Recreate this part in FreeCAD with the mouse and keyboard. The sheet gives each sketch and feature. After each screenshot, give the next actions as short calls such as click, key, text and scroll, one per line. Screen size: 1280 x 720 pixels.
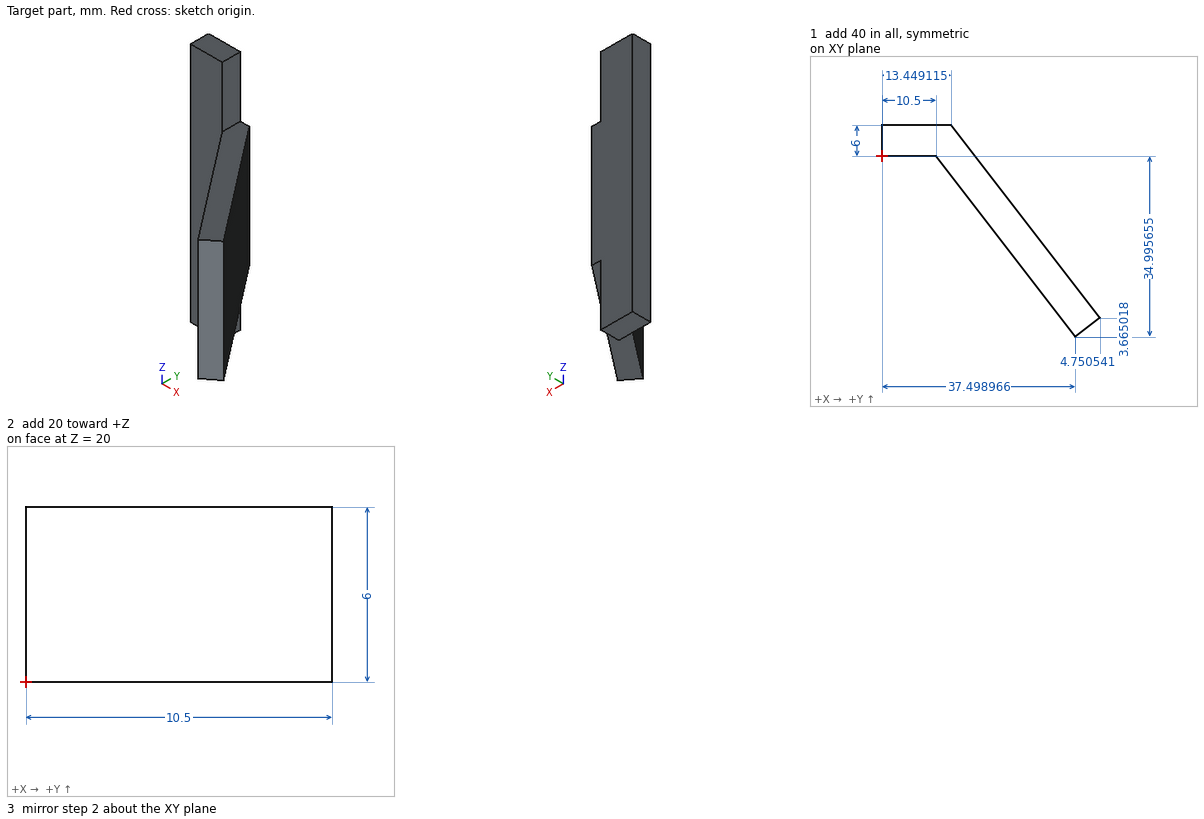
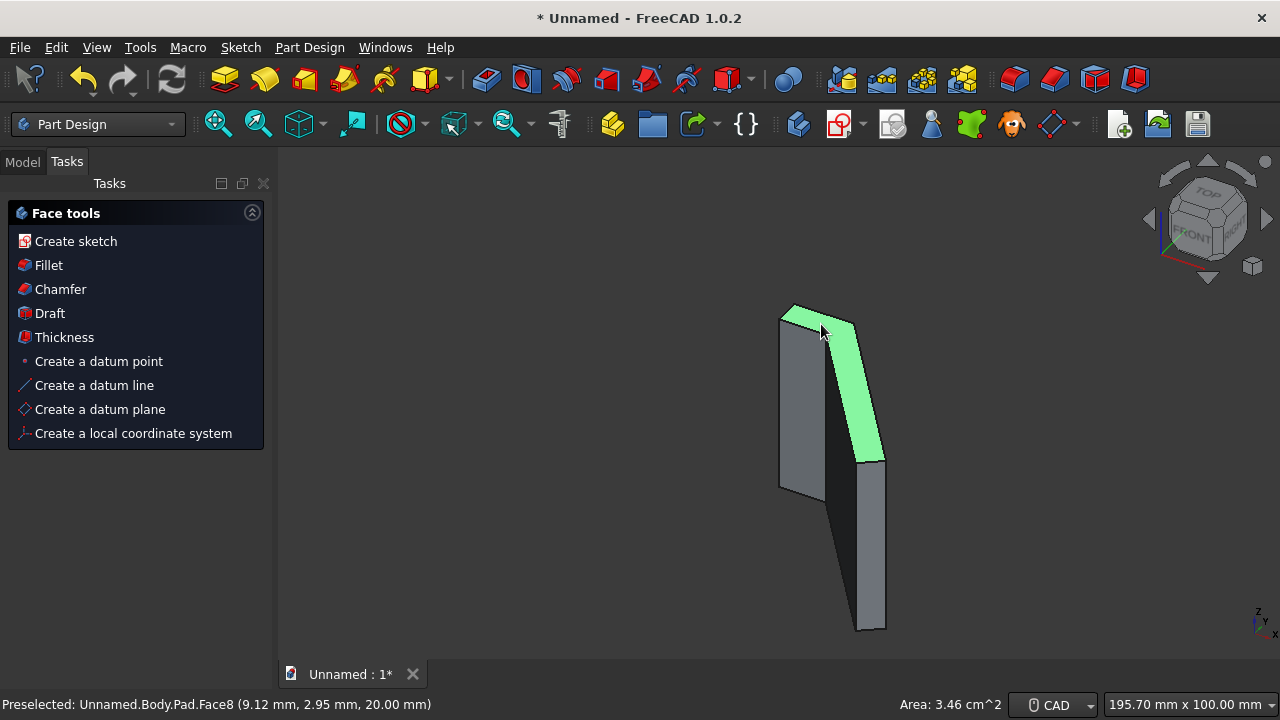
click(840, 124)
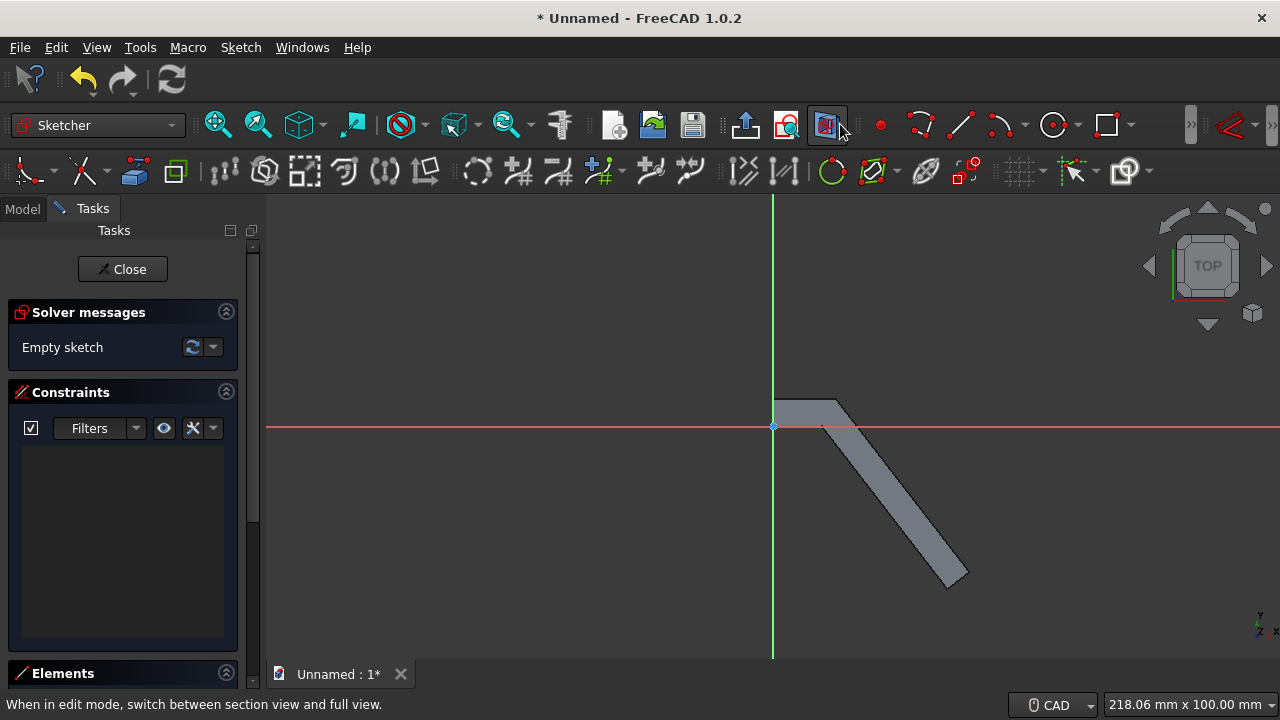
scroll(807, 411, up, 12)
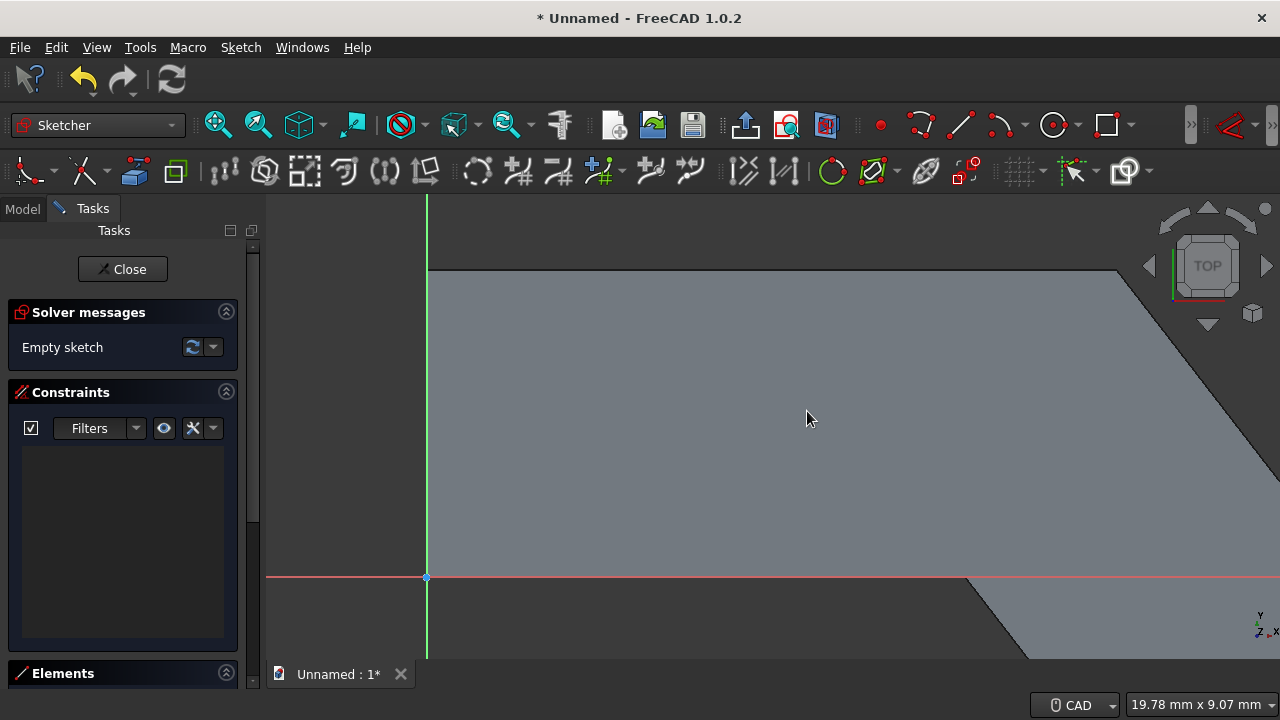
click(1108, 126)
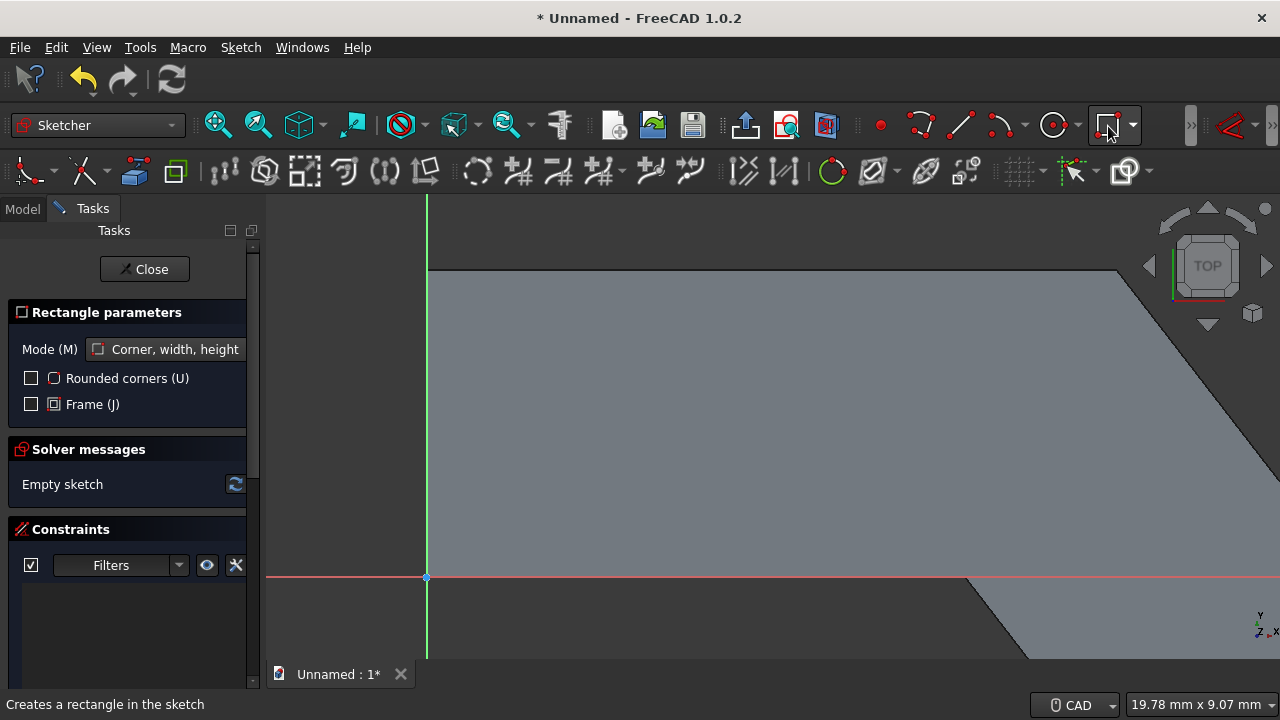
click(427, 577)
click(965, 270)
key(Escape)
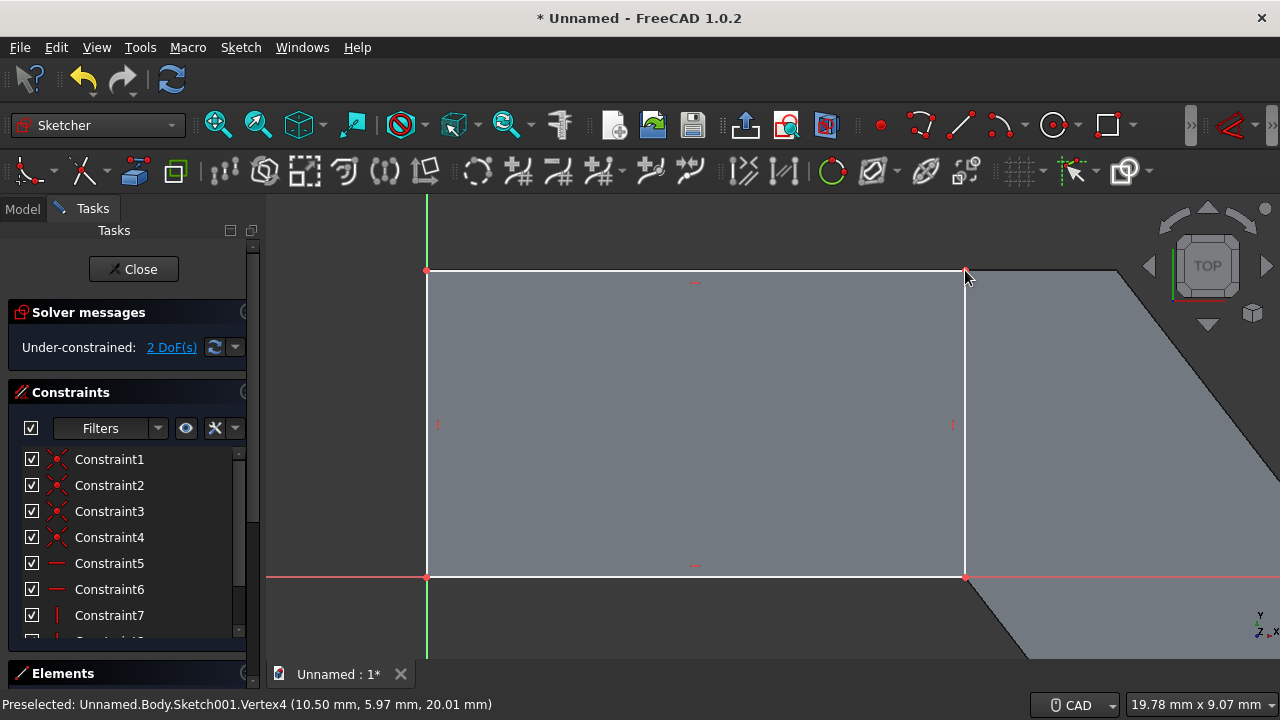
click(1230, 126)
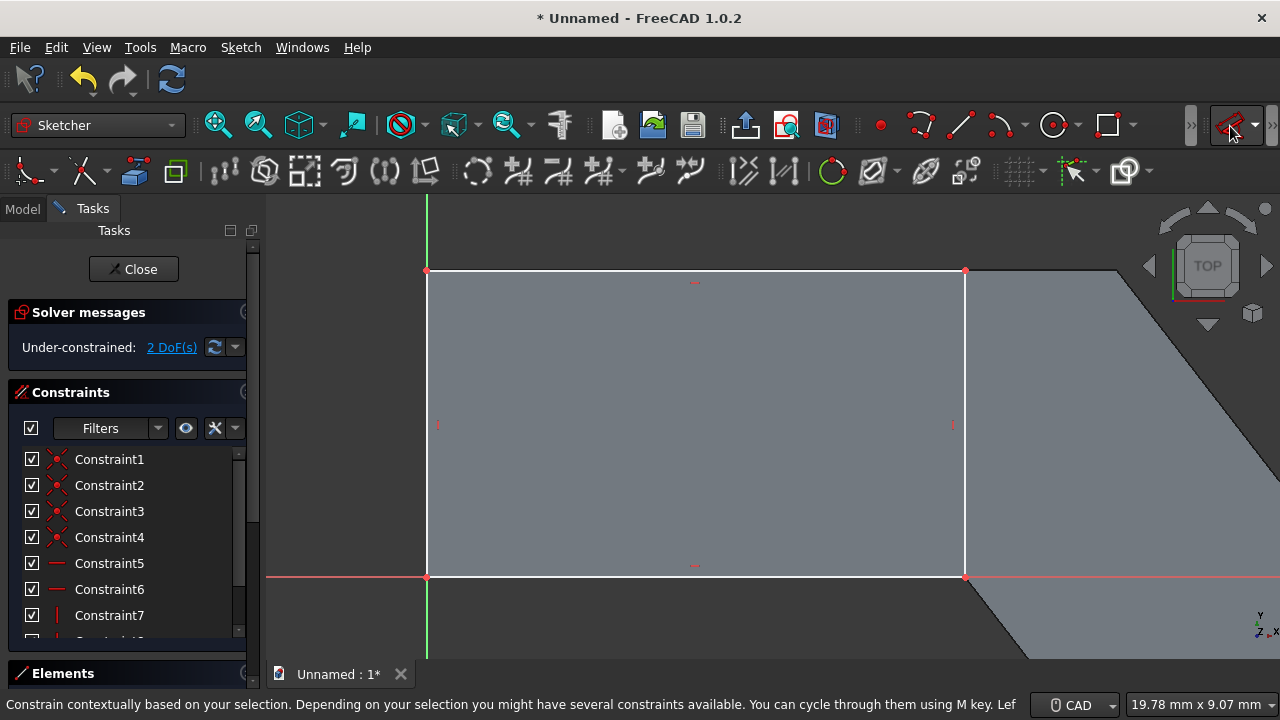
click(965, 485)
click(999, 424)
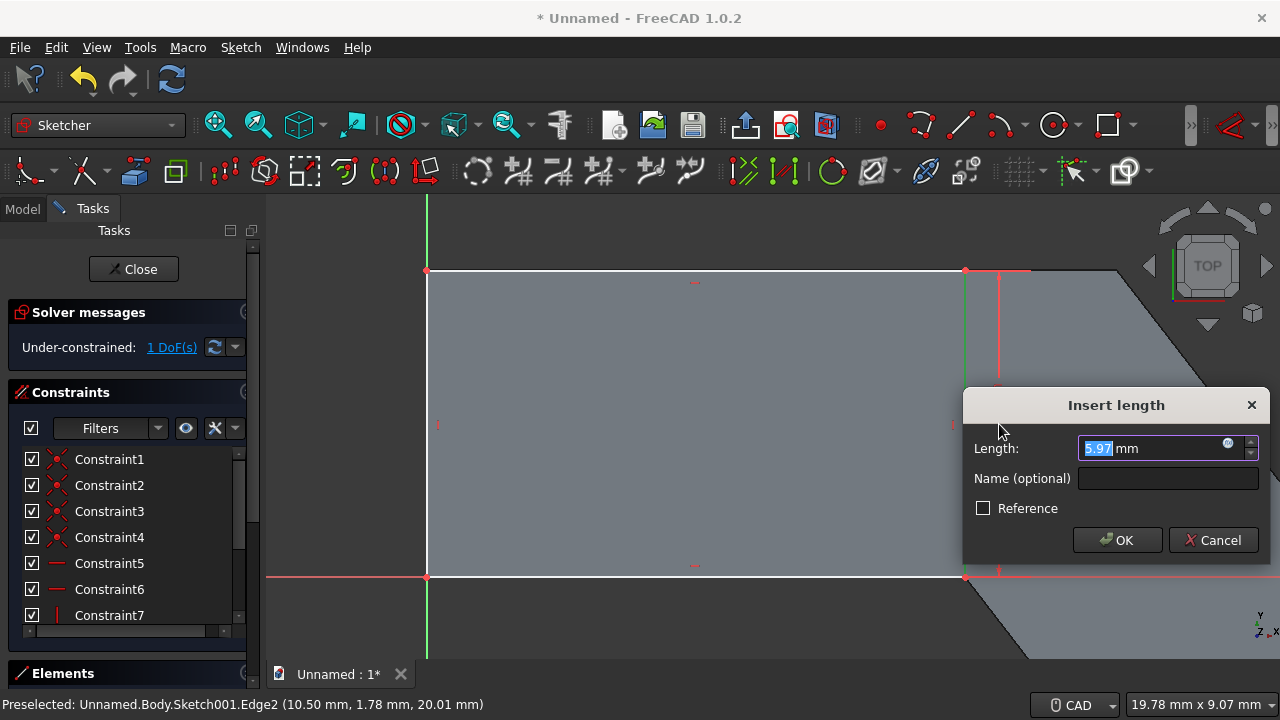
text(6)
key(Return)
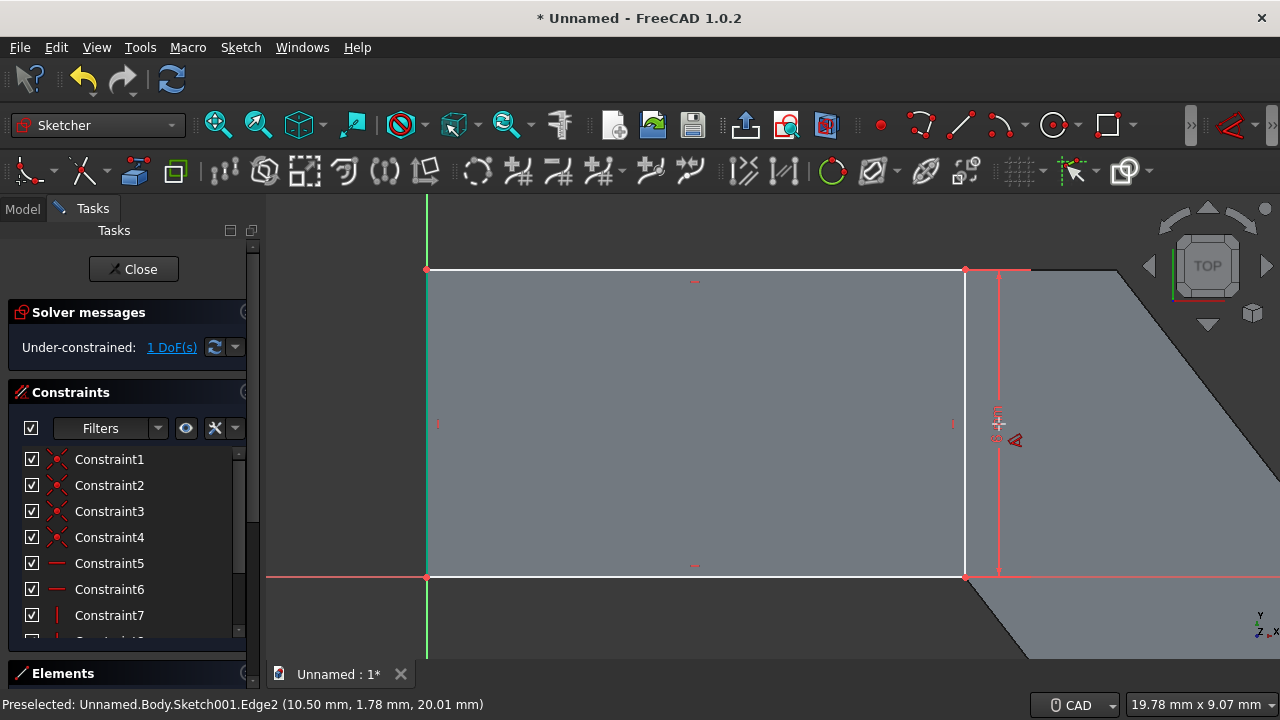
click(588, 577)
click(696, 611)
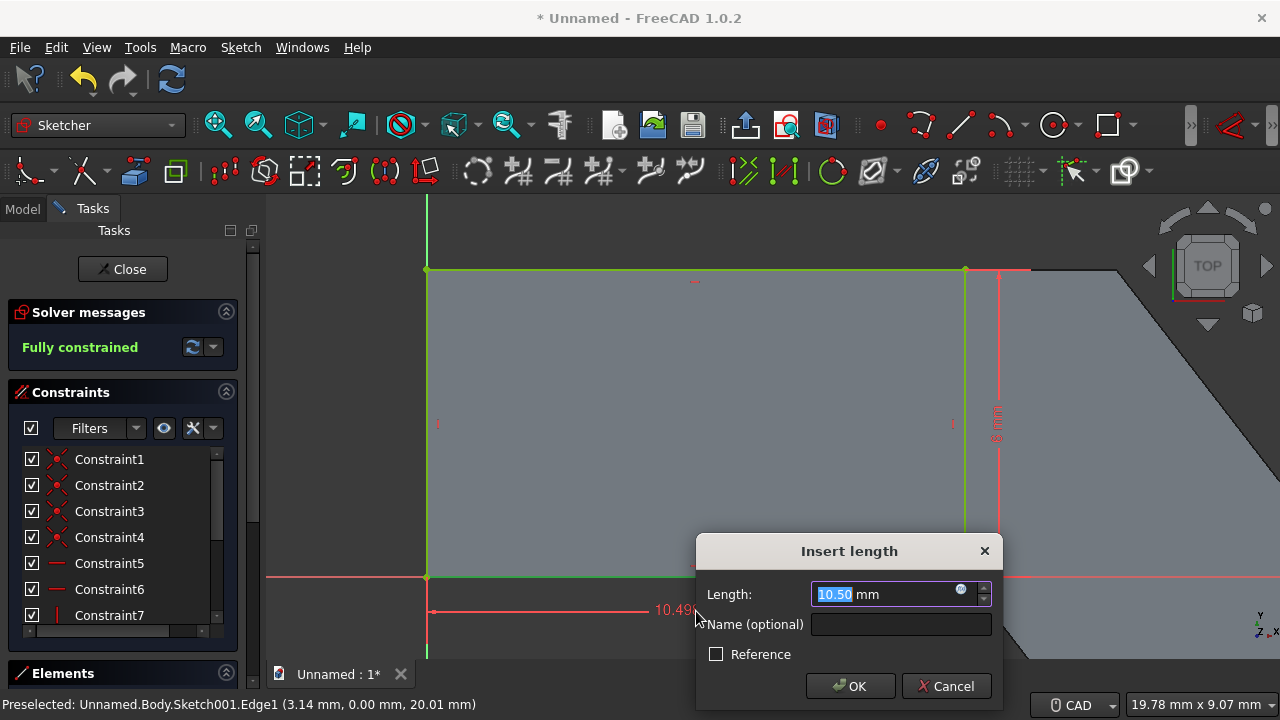
text(10.5)
key(Return)
key(Escape)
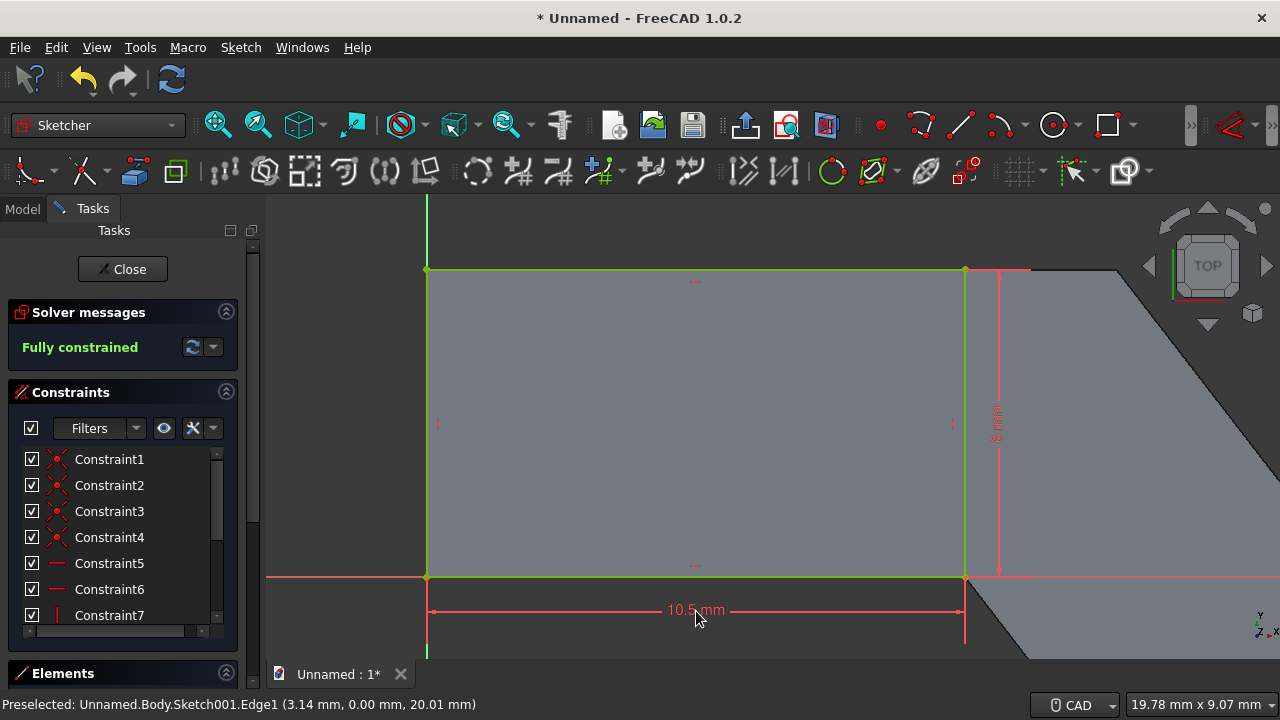
click(123, 269)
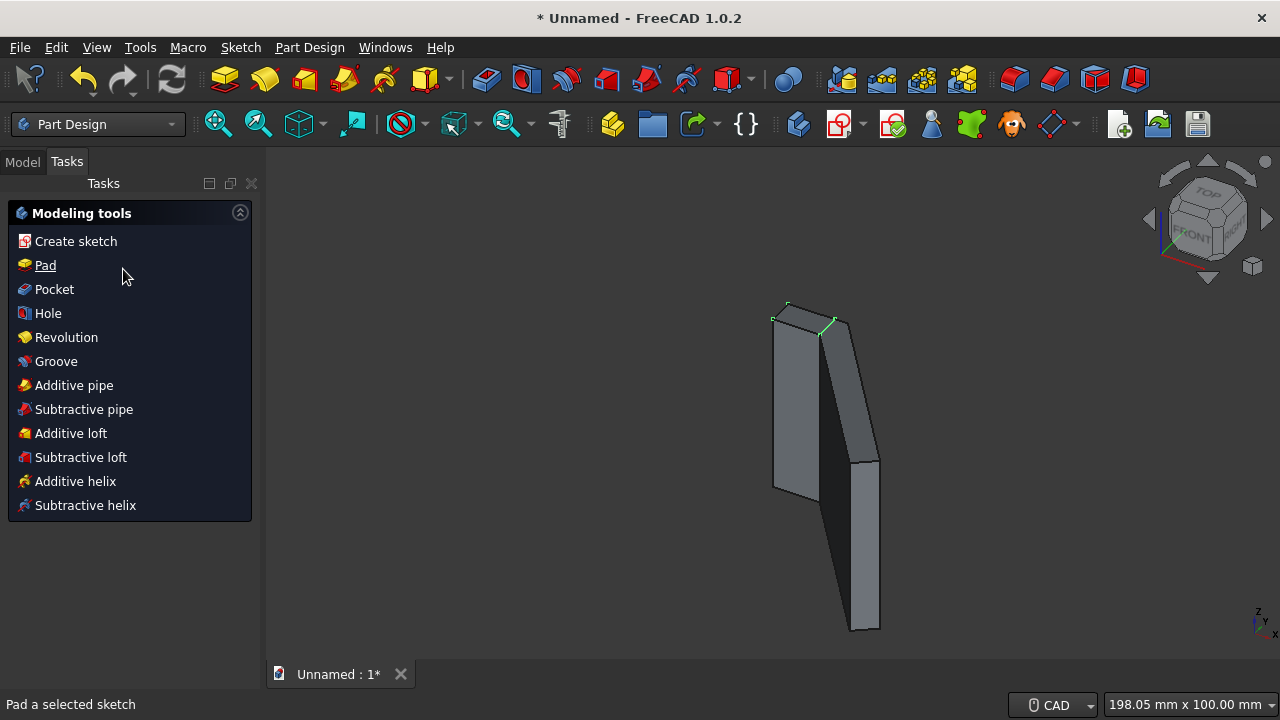
click(226, 80)